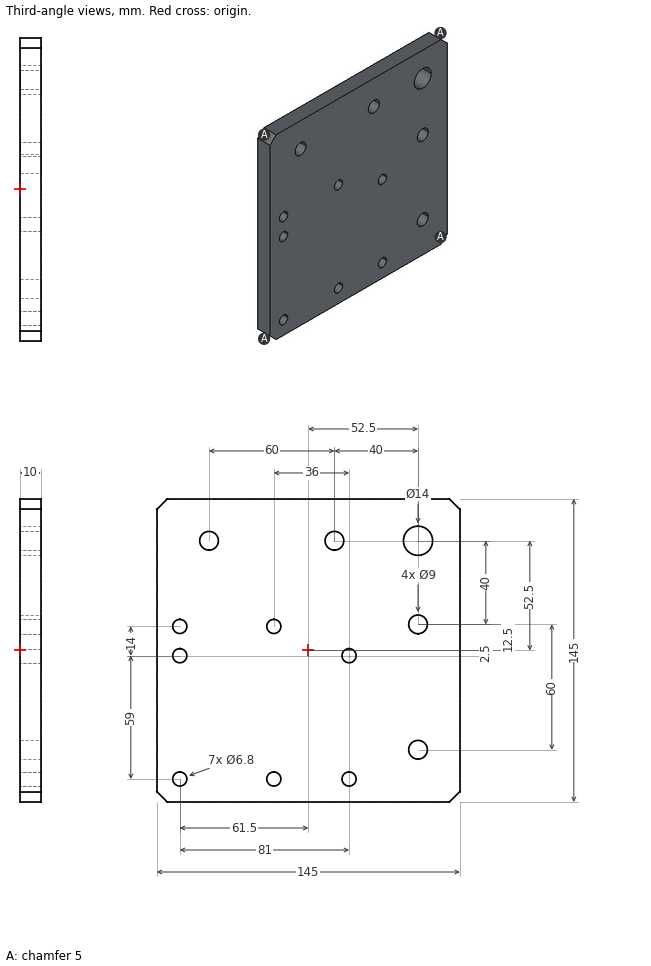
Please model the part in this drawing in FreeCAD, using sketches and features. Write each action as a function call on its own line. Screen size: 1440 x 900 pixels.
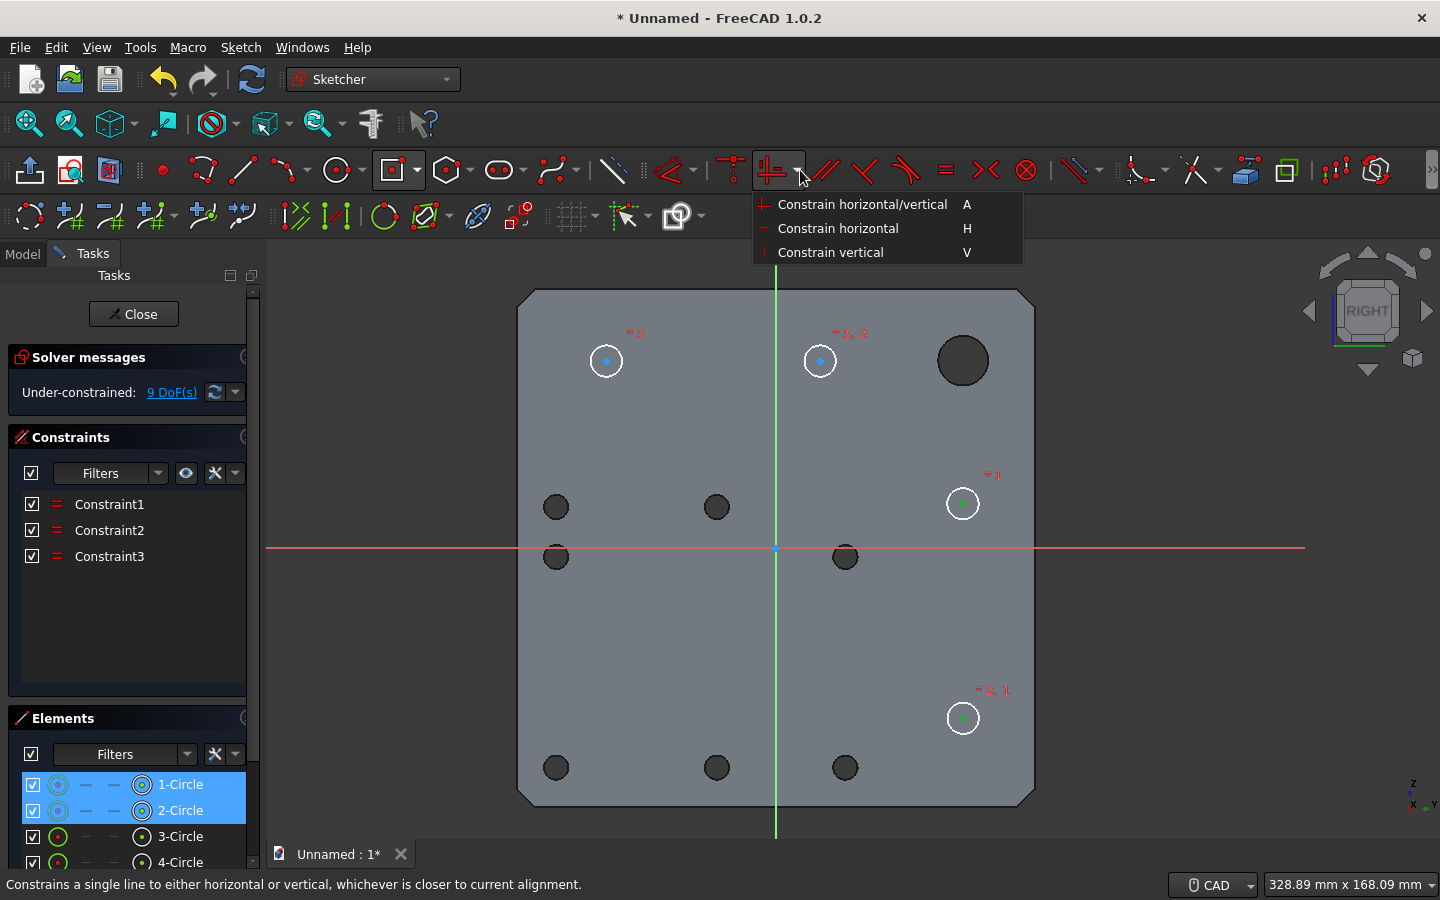
click(888, 252)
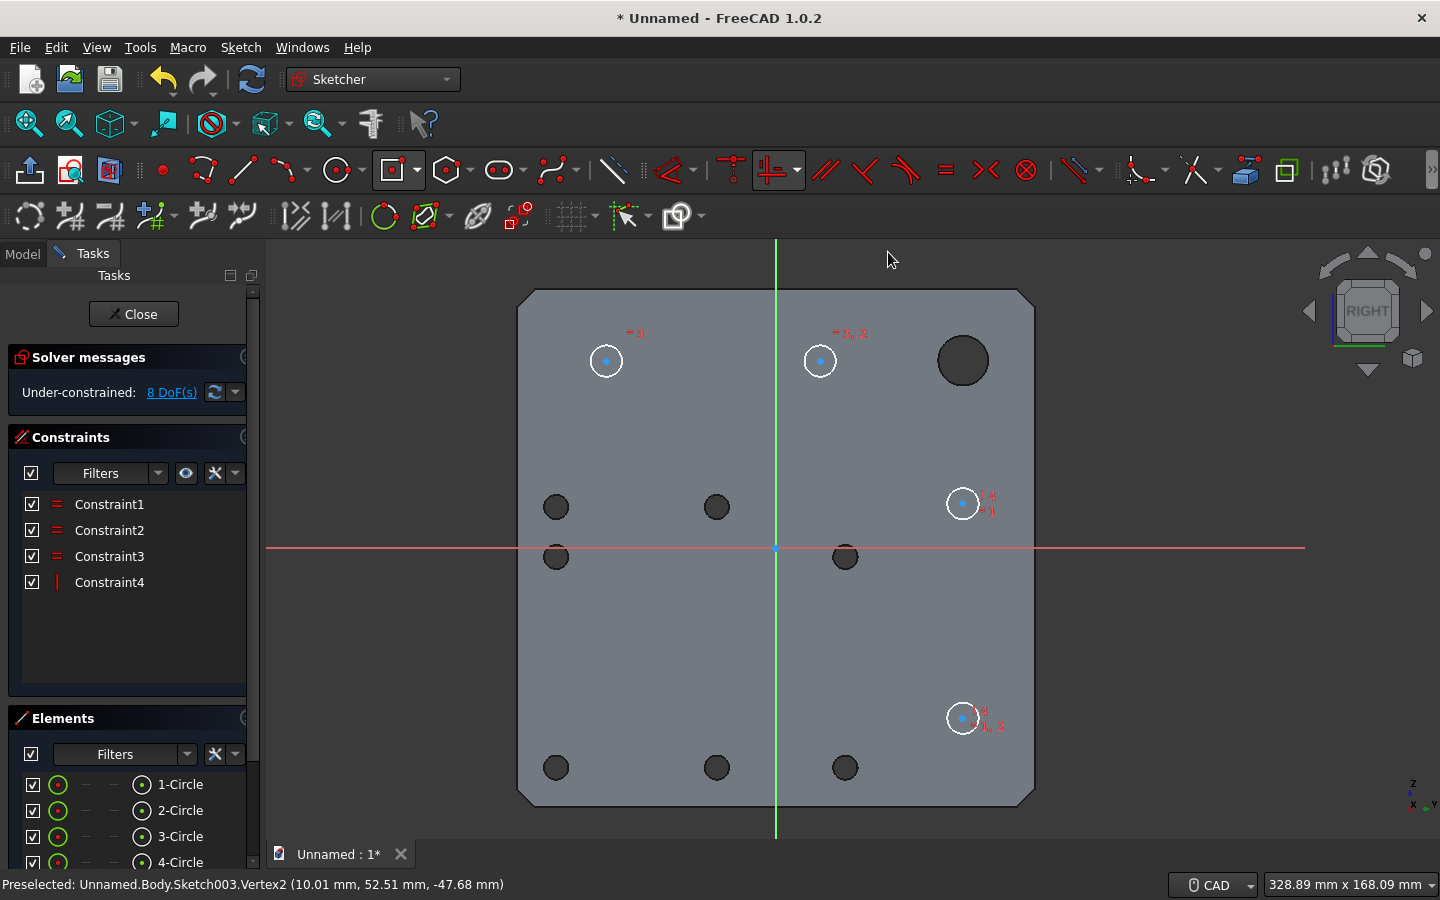
click(820, 361)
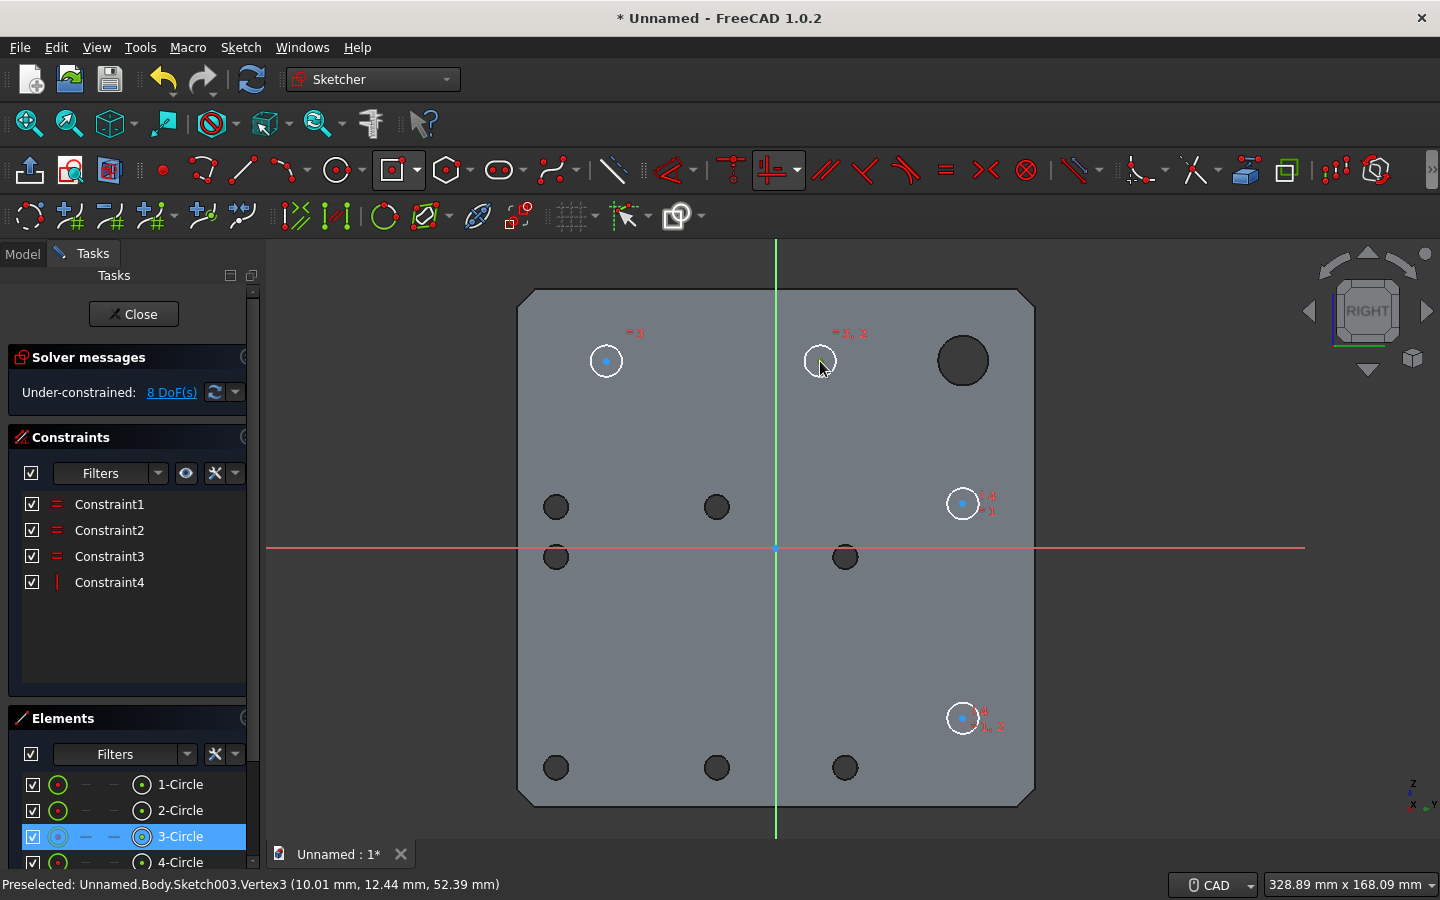
click(606, 361)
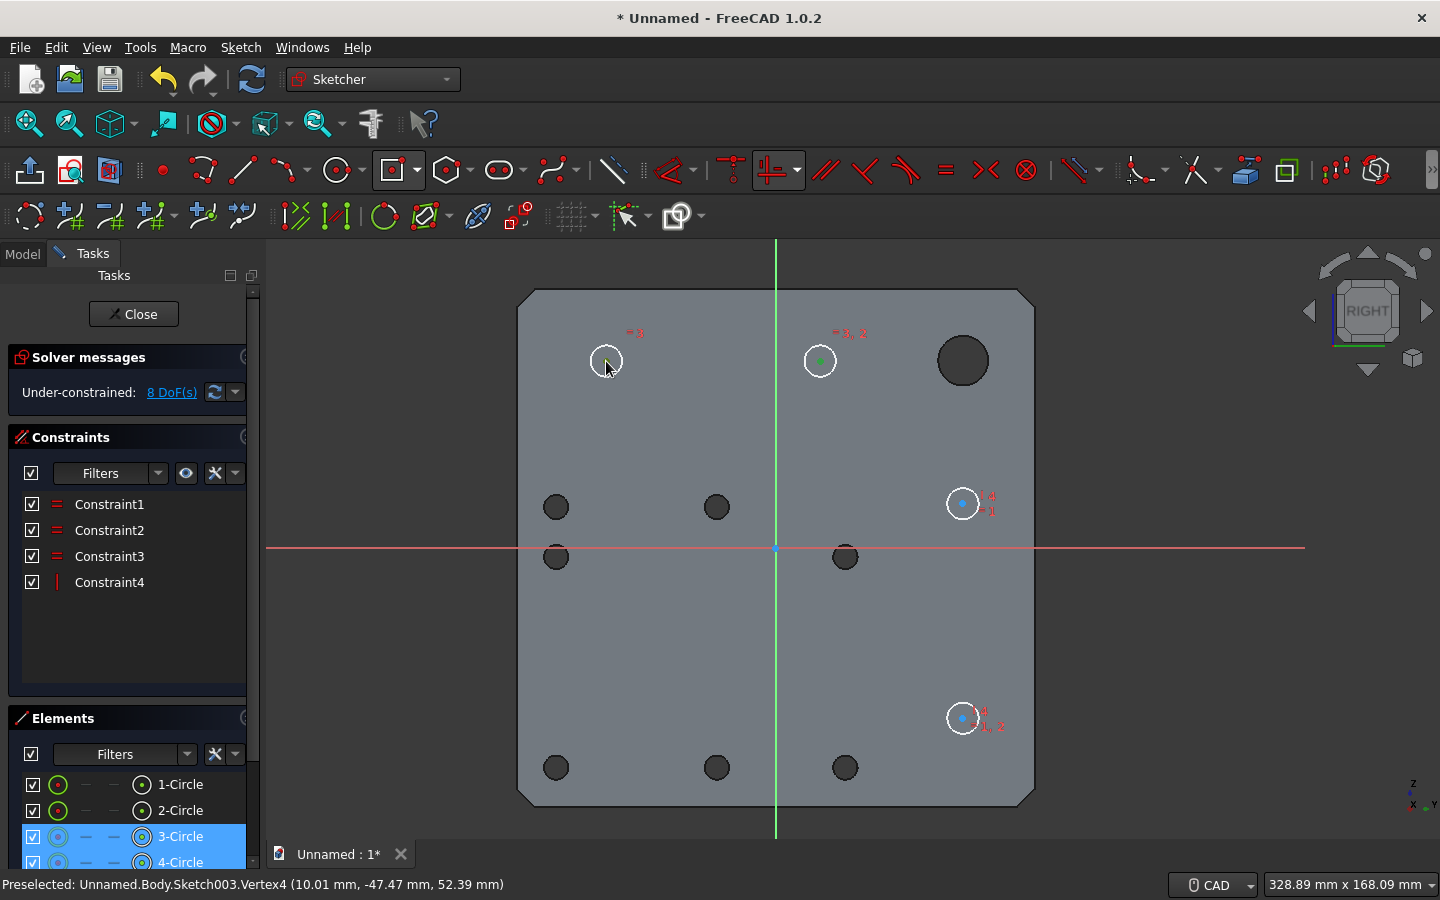
click(800, 170)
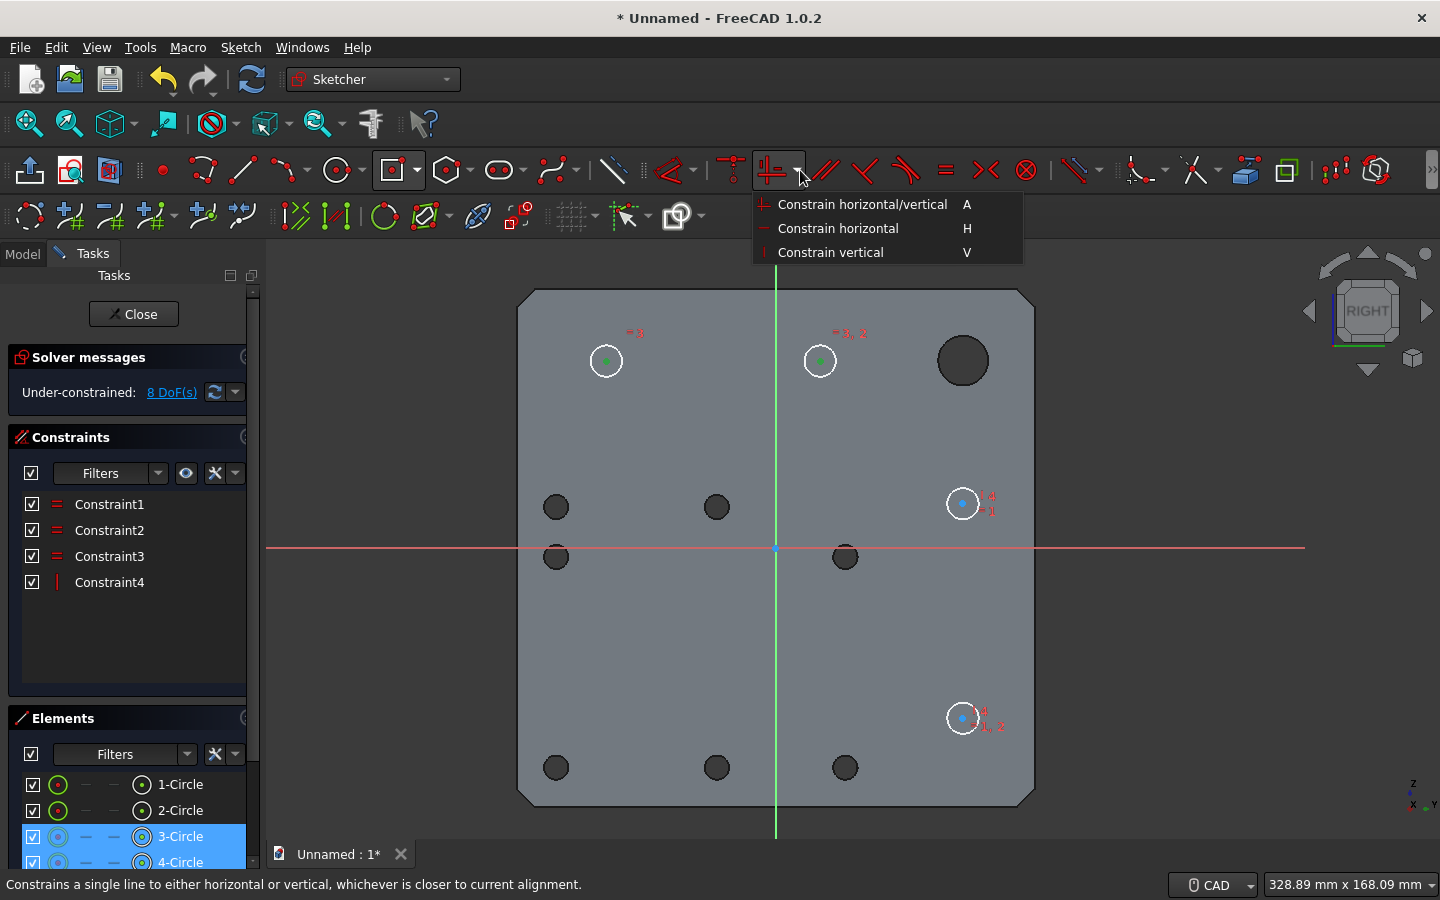
click(888, 228)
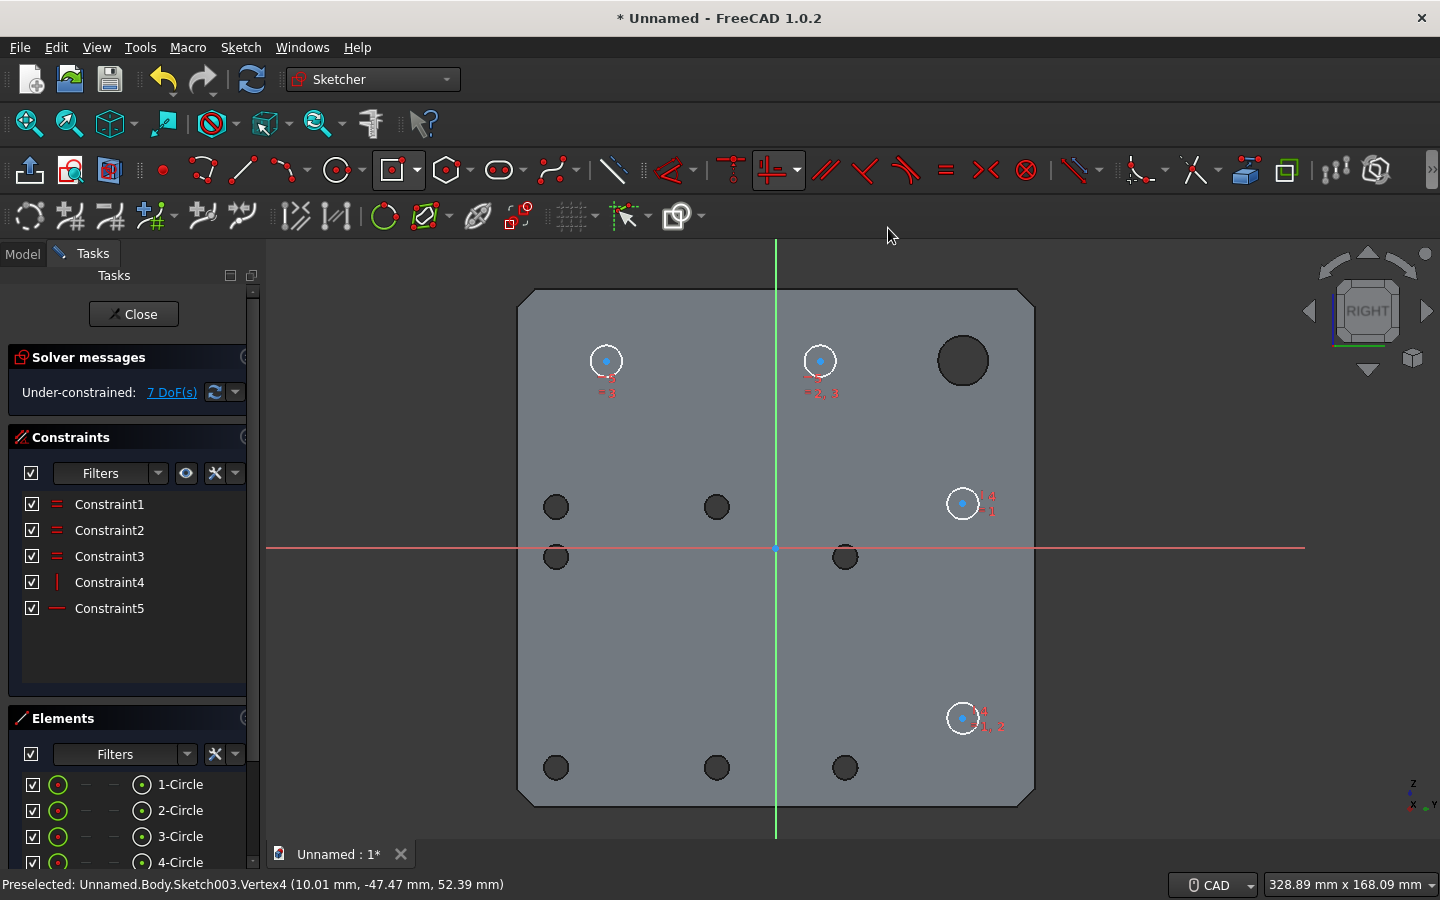
click(668, 170)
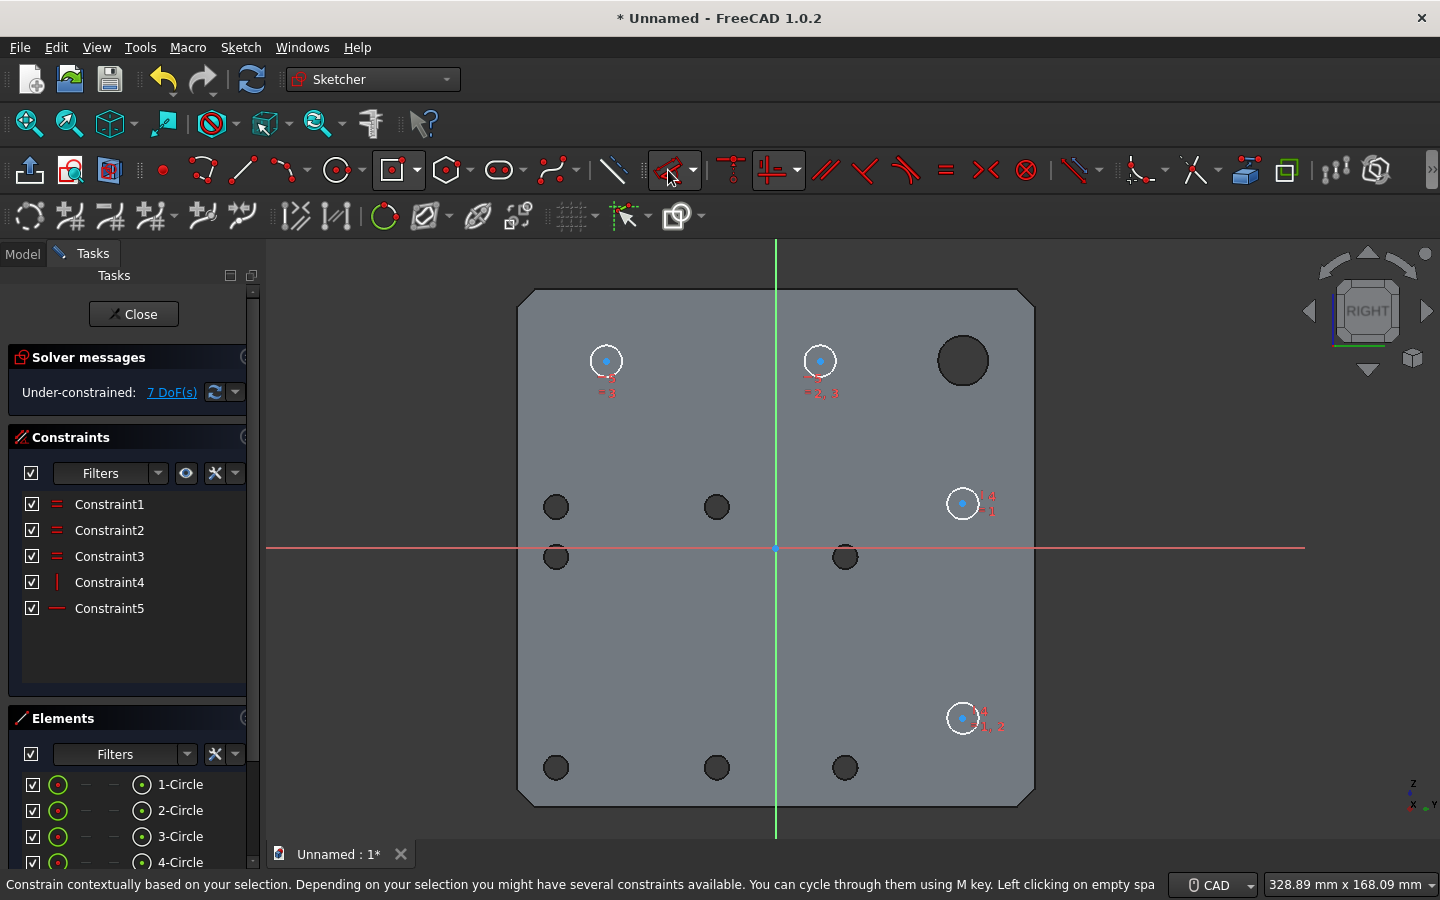
scroll(974, 493, up, 2)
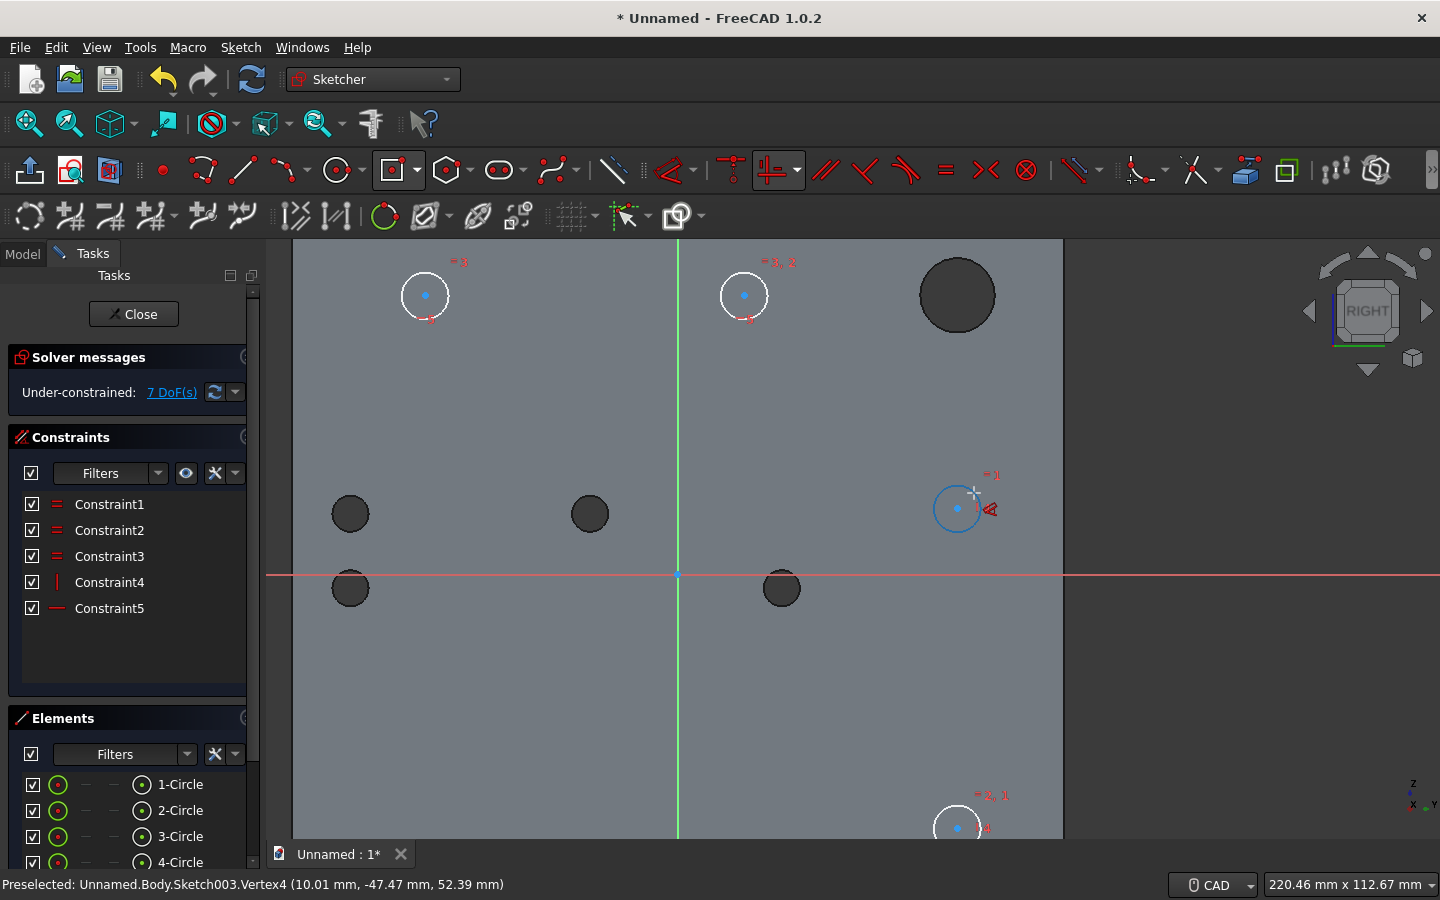
click(974, 492)
click(997, 469)